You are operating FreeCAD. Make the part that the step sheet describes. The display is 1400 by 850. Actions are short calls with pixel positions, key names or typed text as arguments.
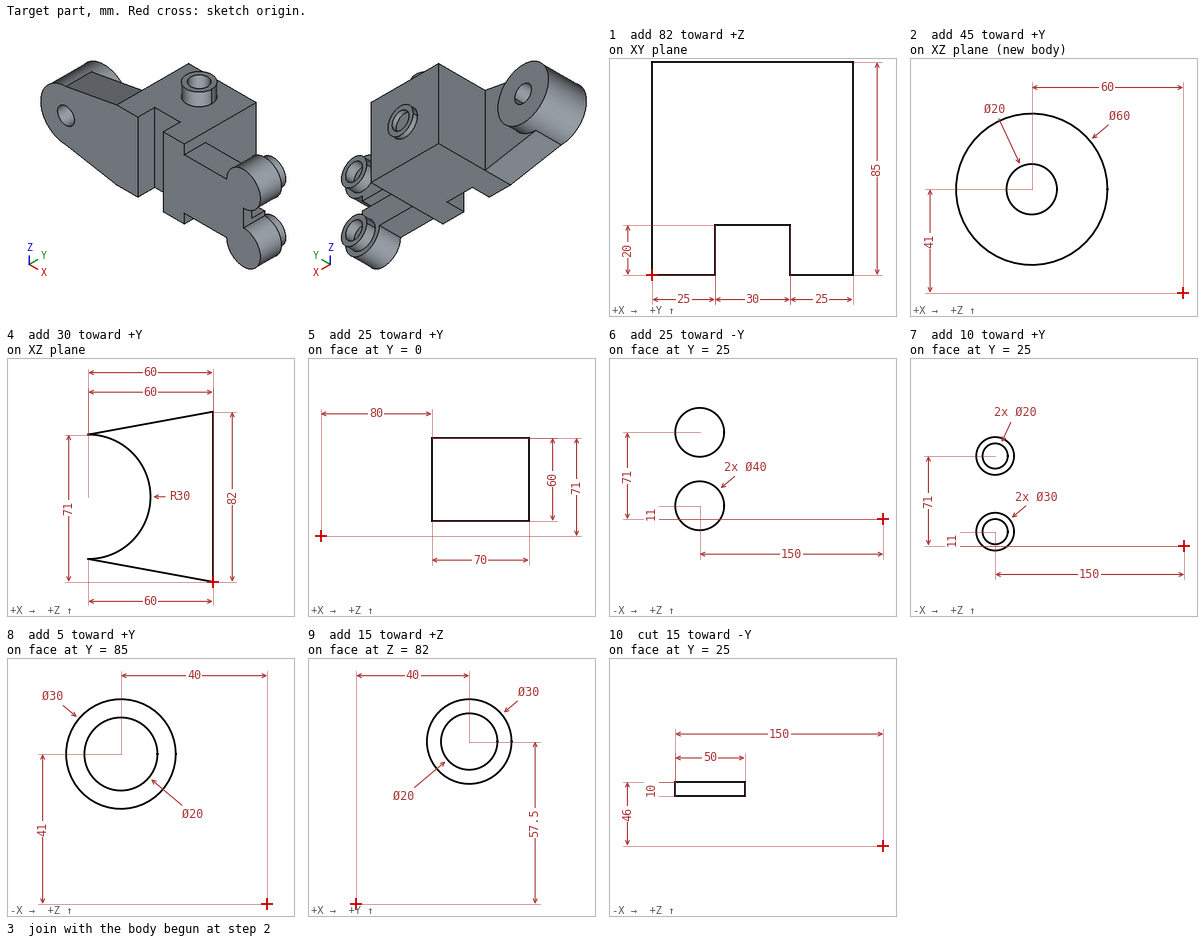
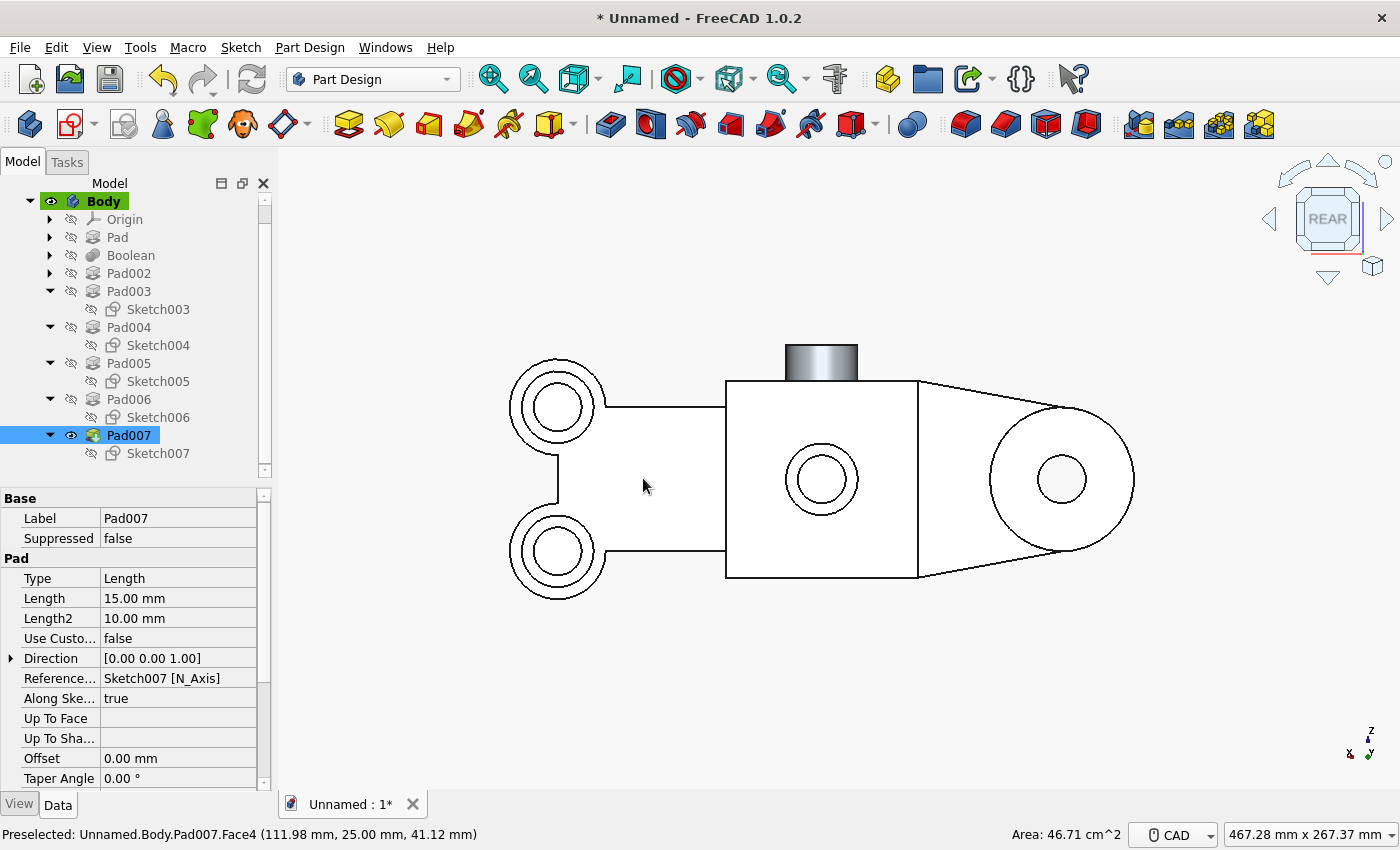
click(70, 124)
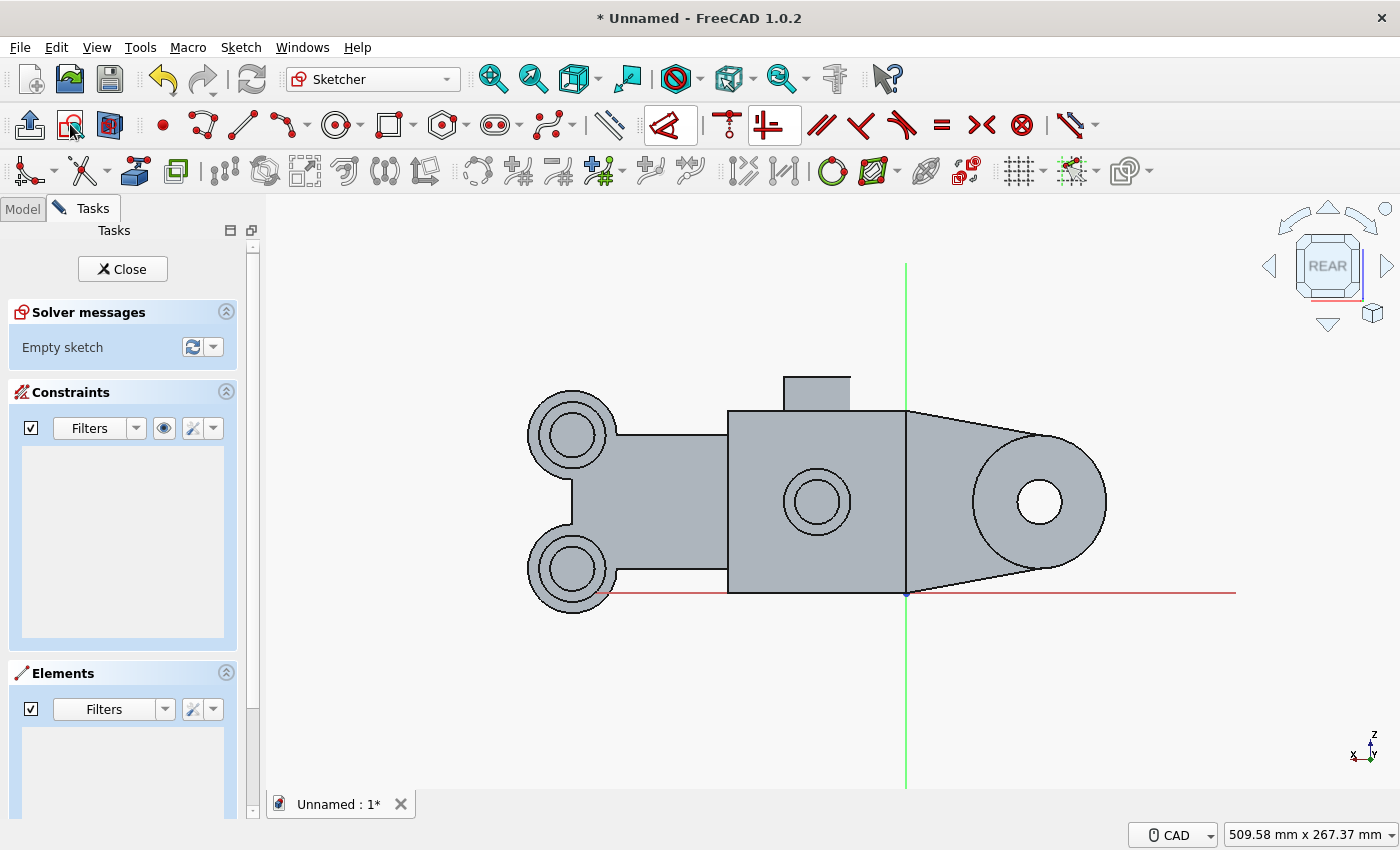
key(q)
key(s)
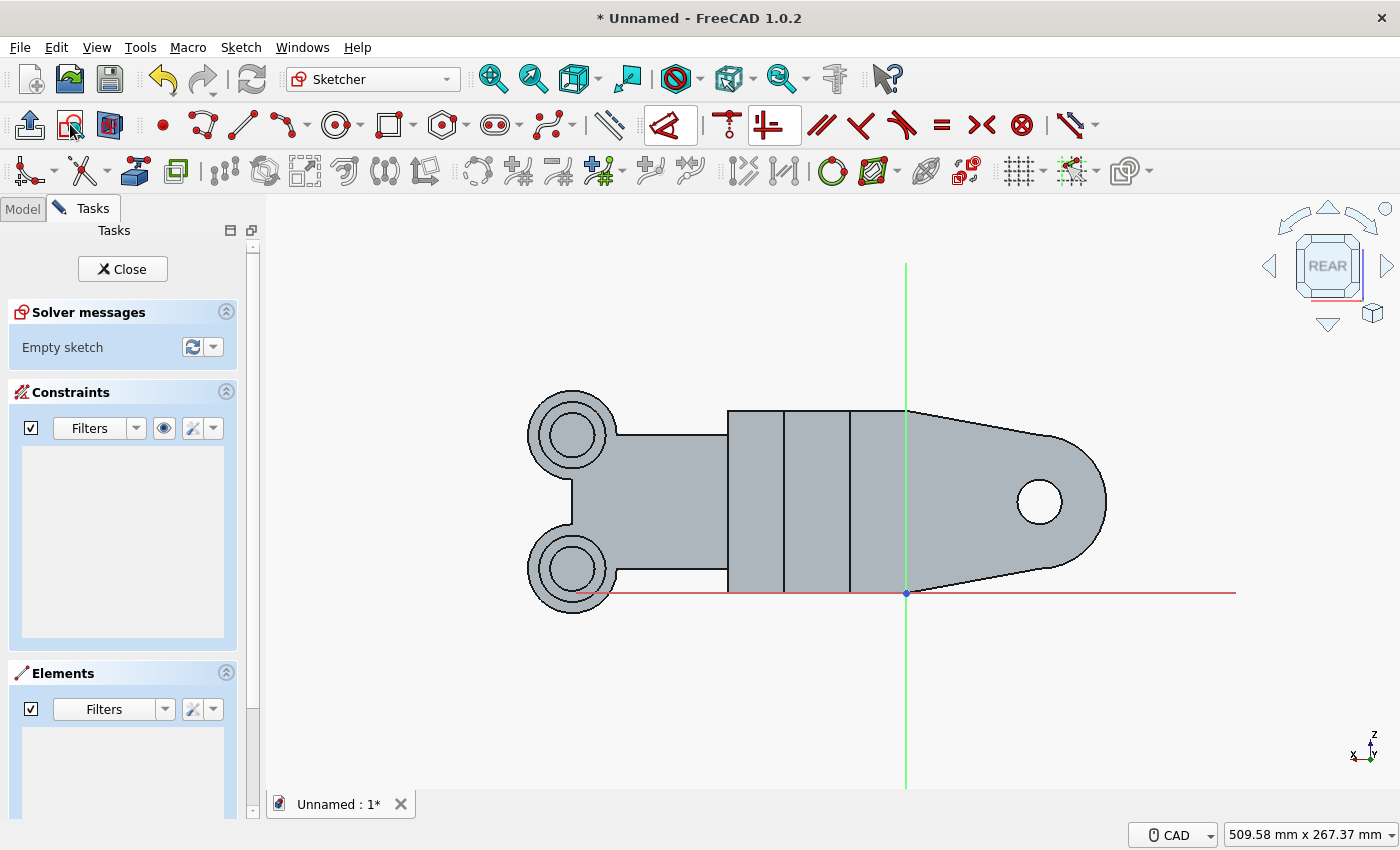
scroll(601, 504, up, 9)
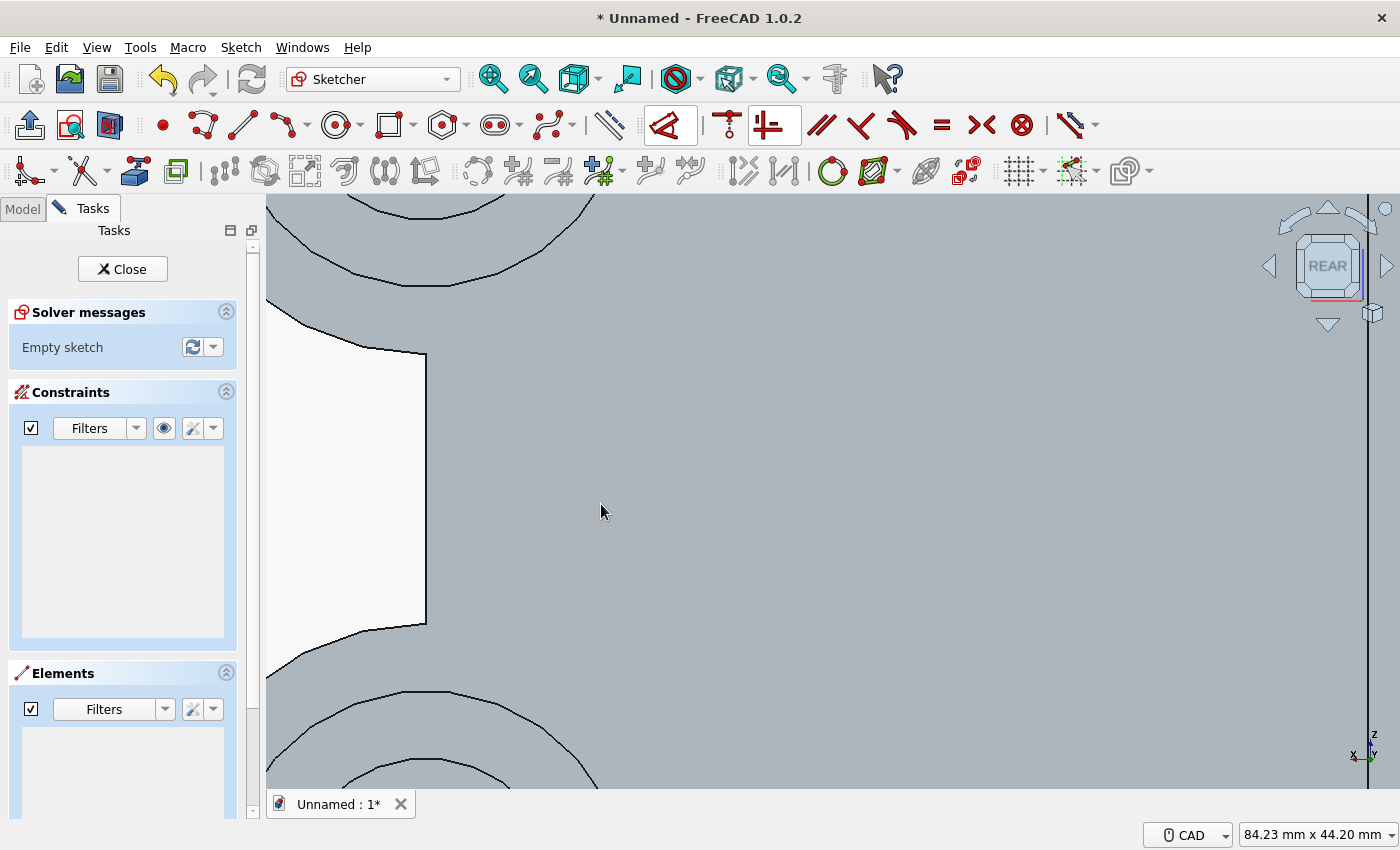
click(390, 126)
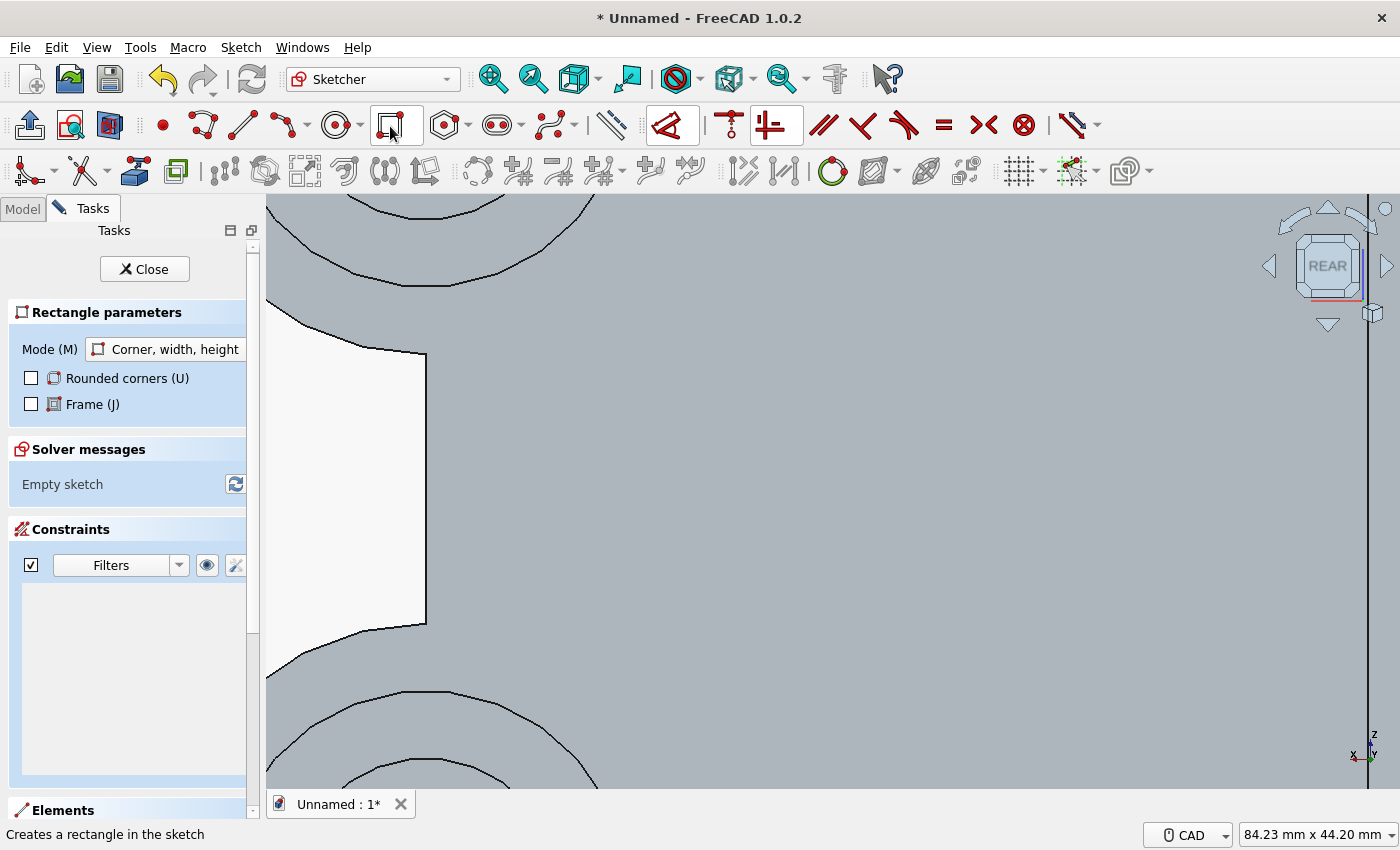
click(426, 422)
click(1099, 556)
key(Escape)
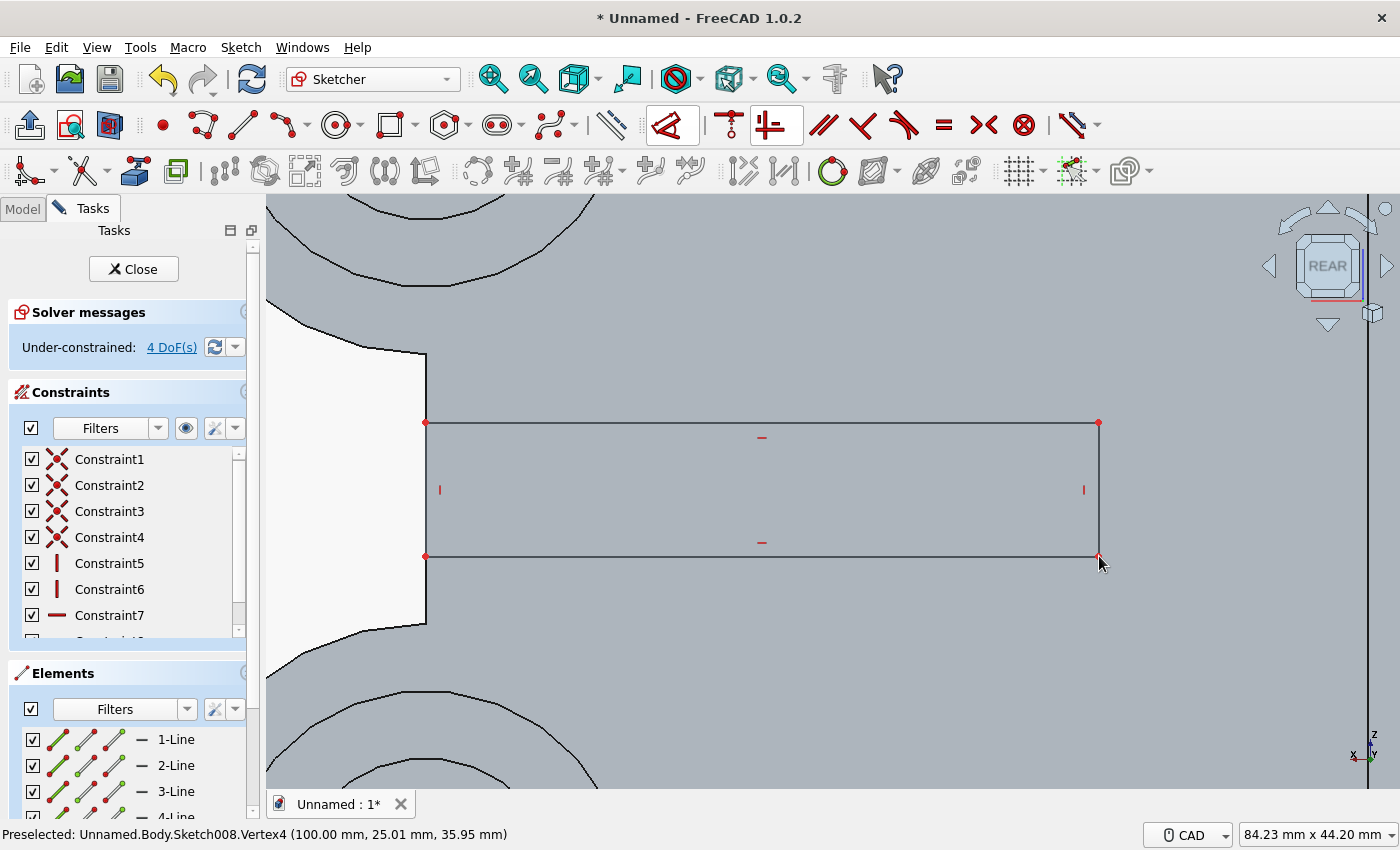
click(426, 463)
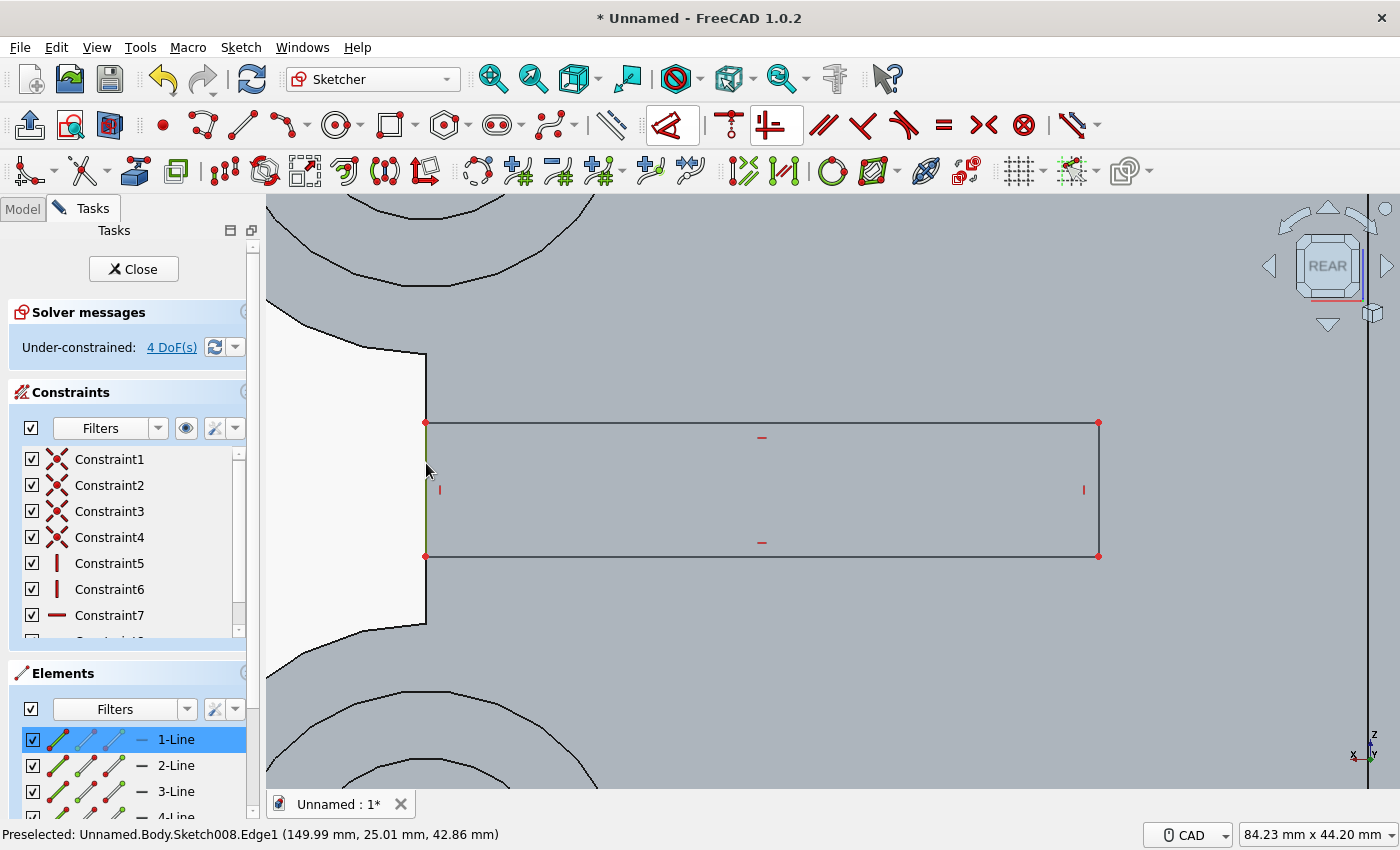
click(694, 126)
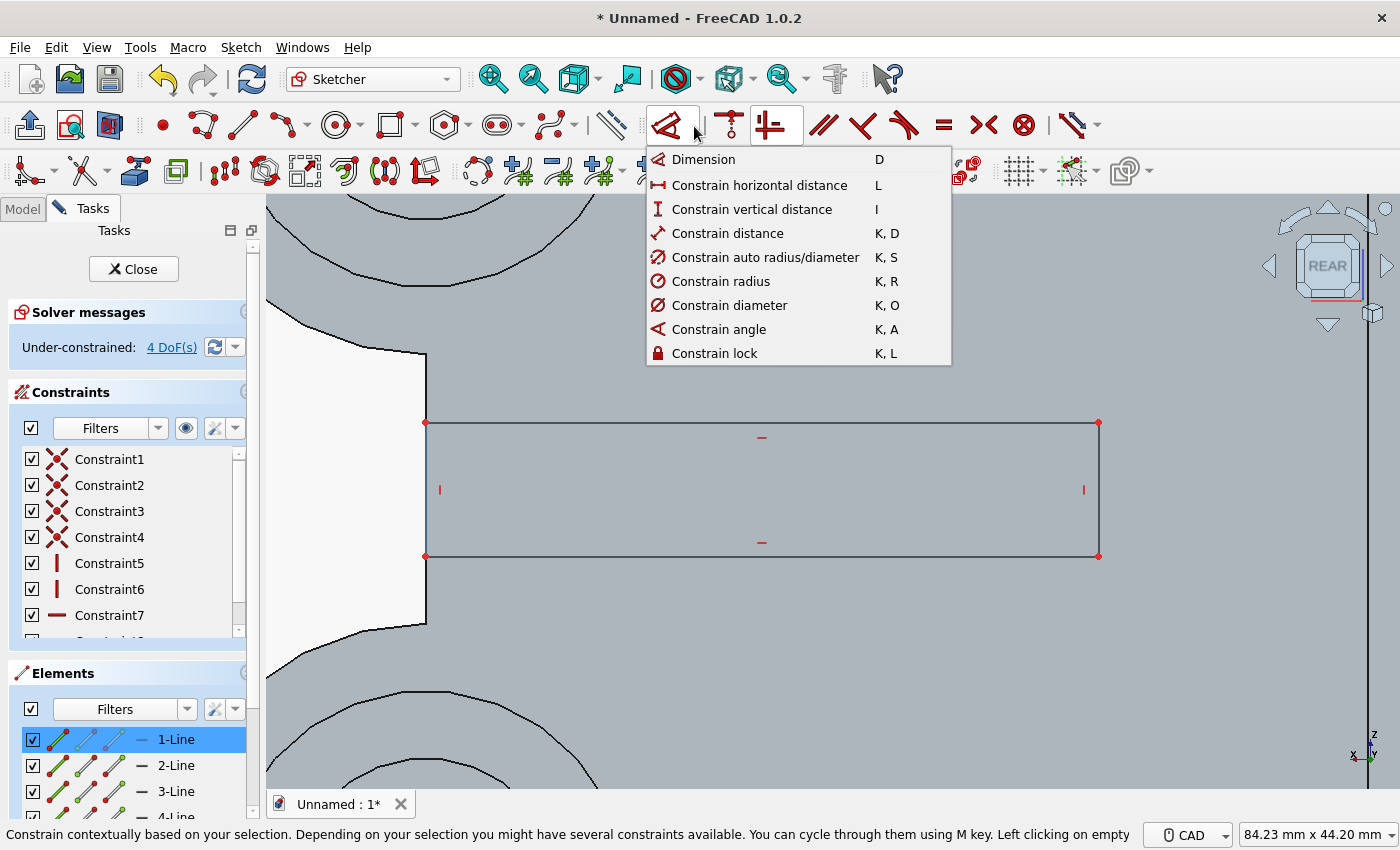
click(799, 209)